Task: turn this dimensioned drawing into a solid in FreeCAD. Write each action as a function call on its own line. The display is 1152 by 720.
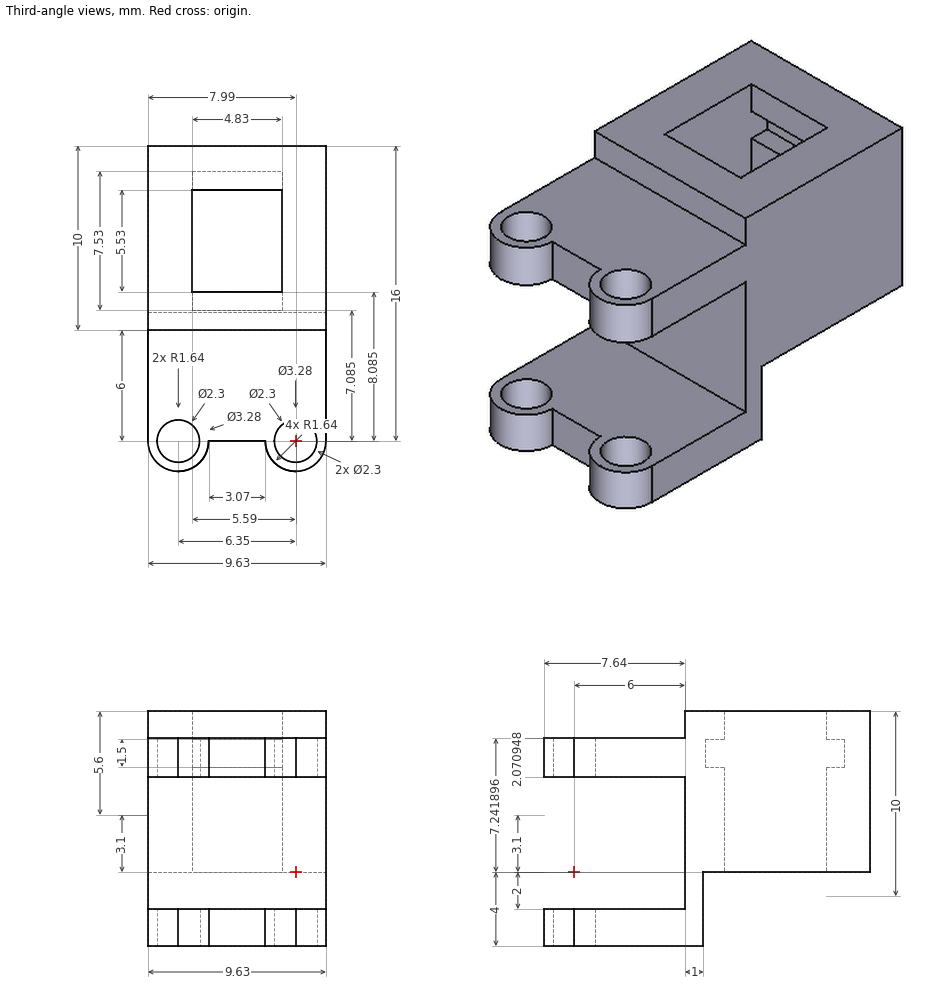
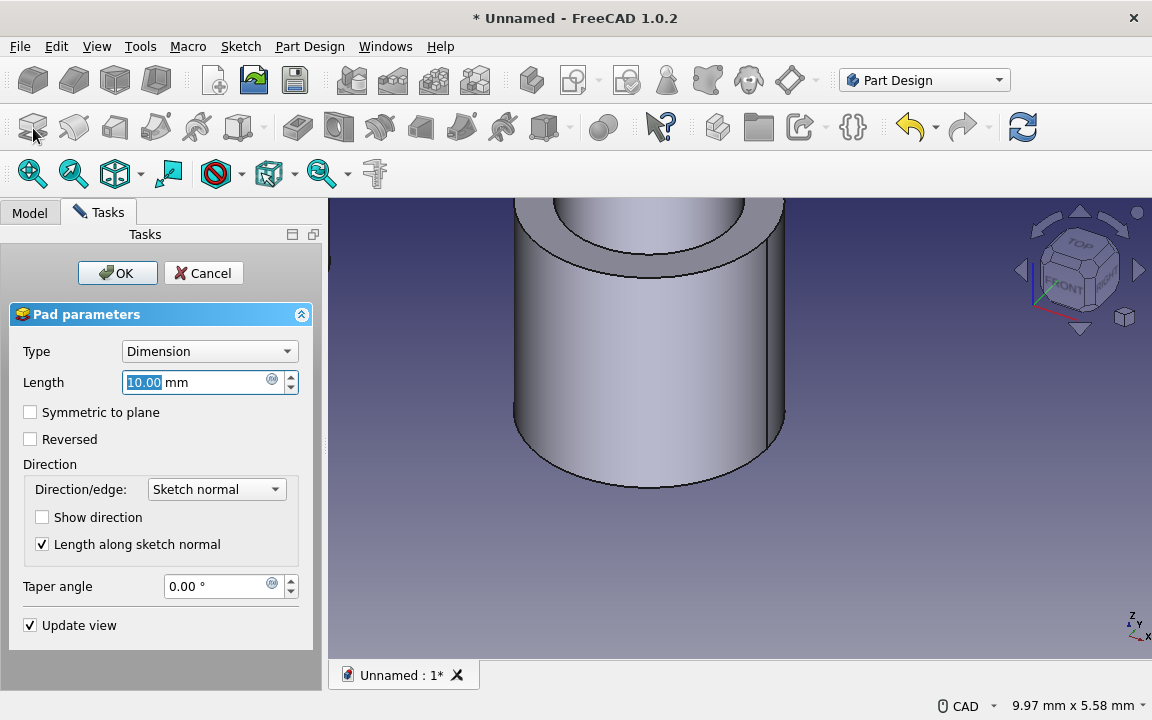
text(3.1)
key(Tab)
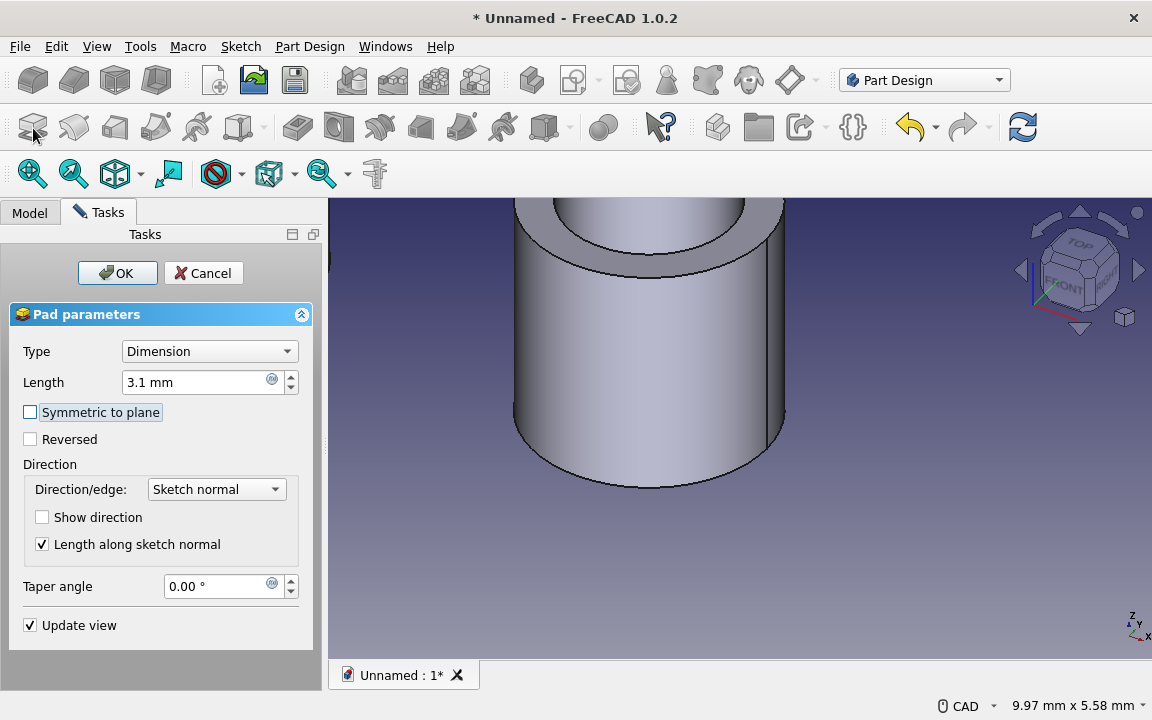
click(118, 273)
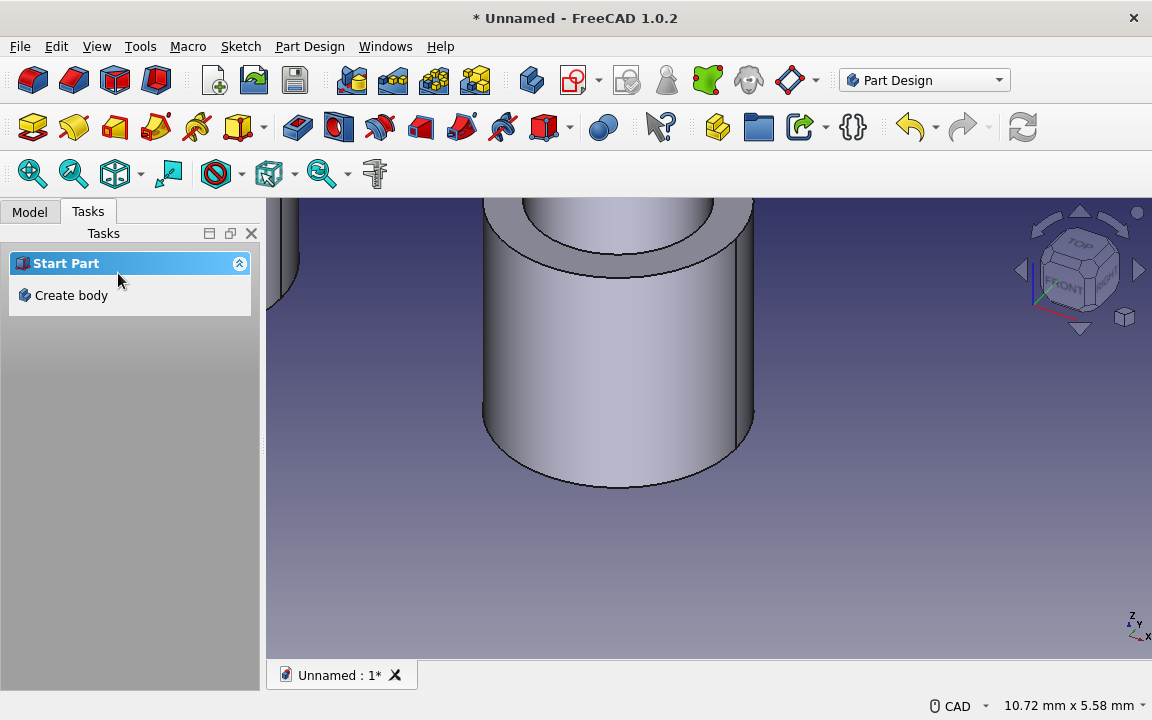
click(33, 174)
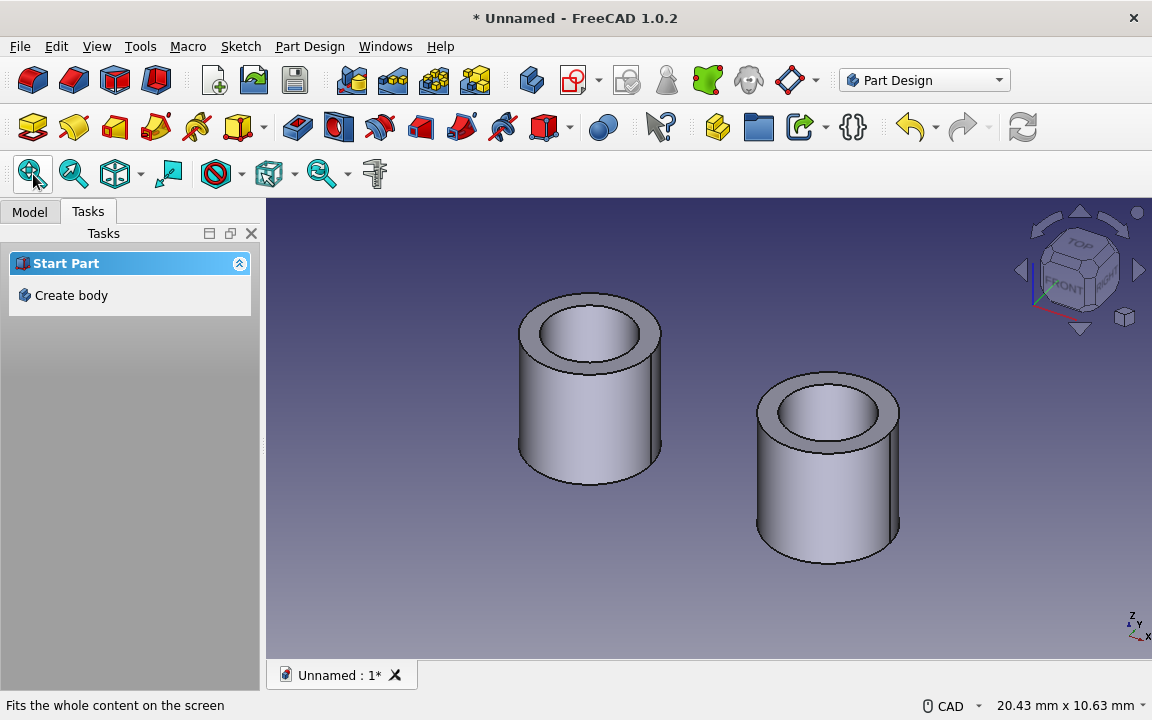
click(30, 212)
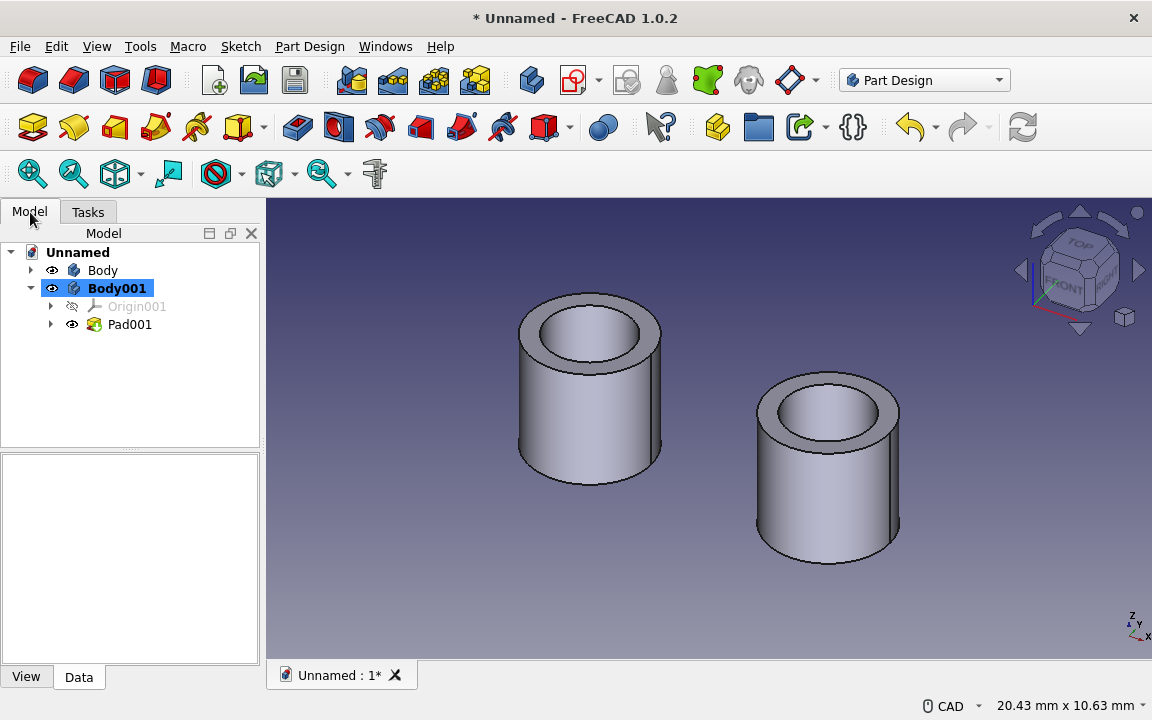
double_click(97, 270)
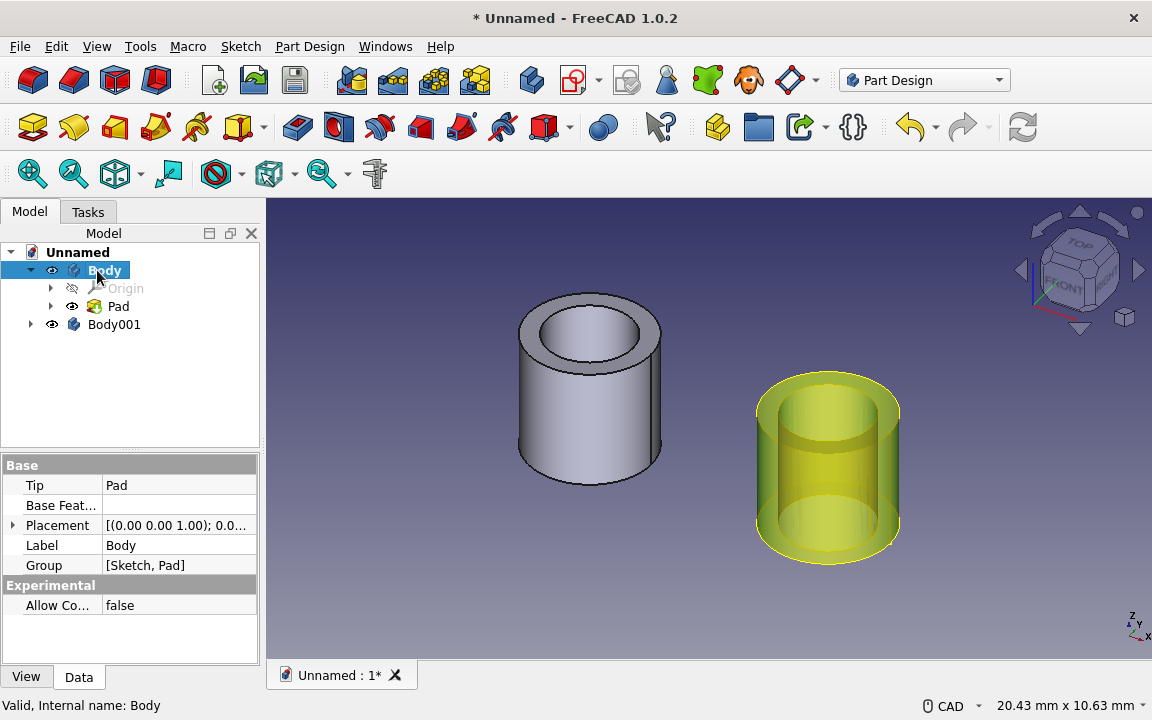
click(97, 270)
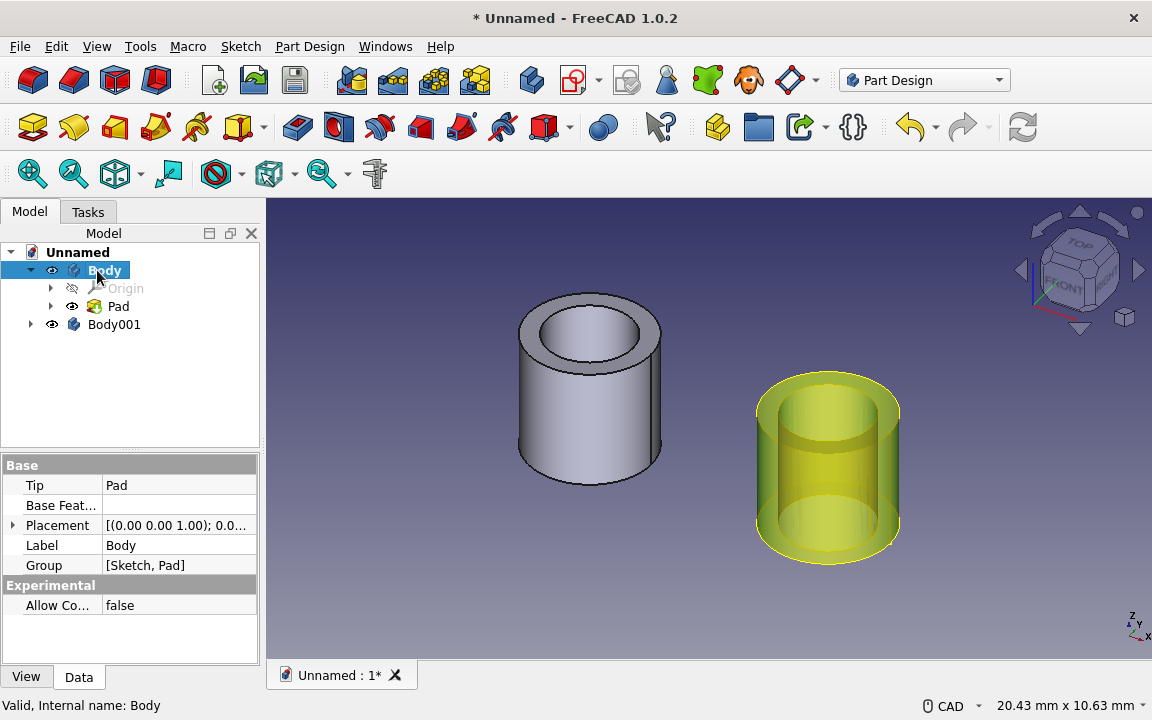
click(148, 605)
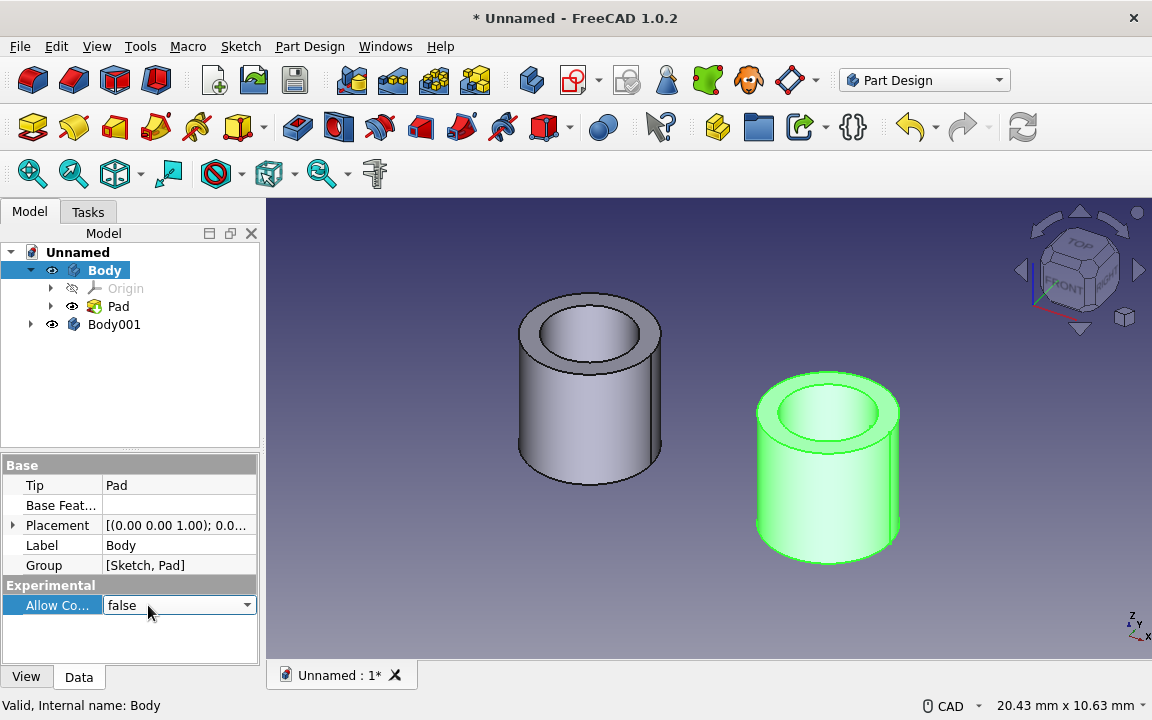
click(148, 605)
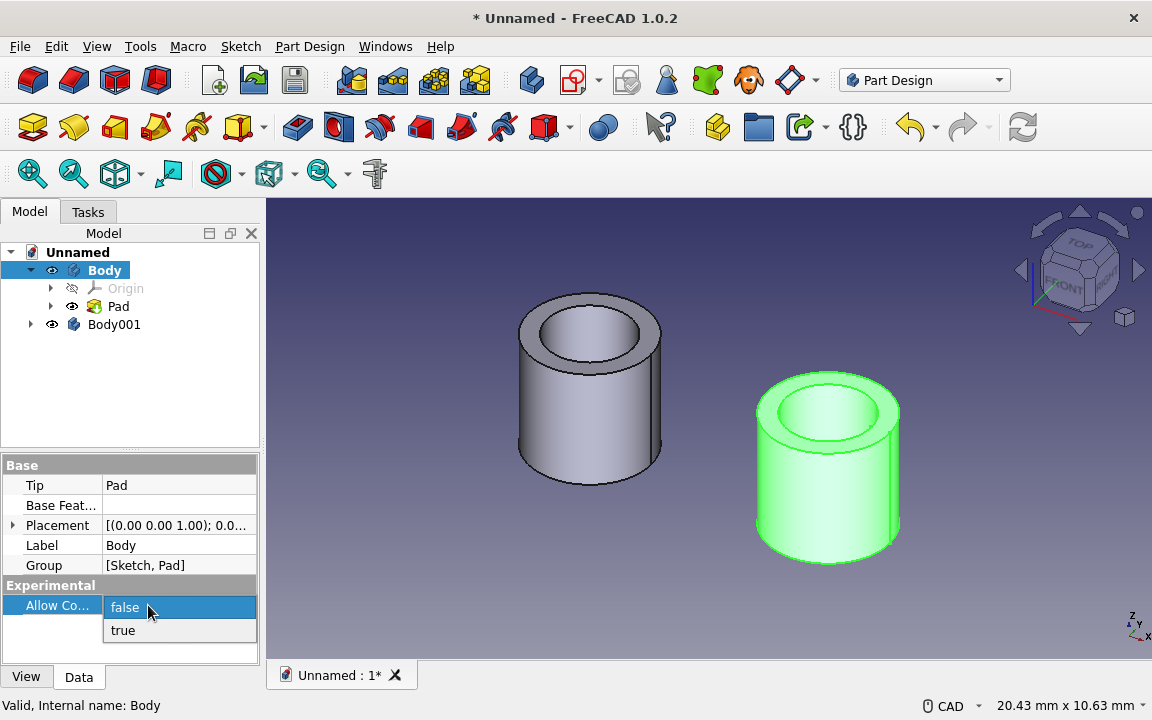
click(178, 630)
key(Return)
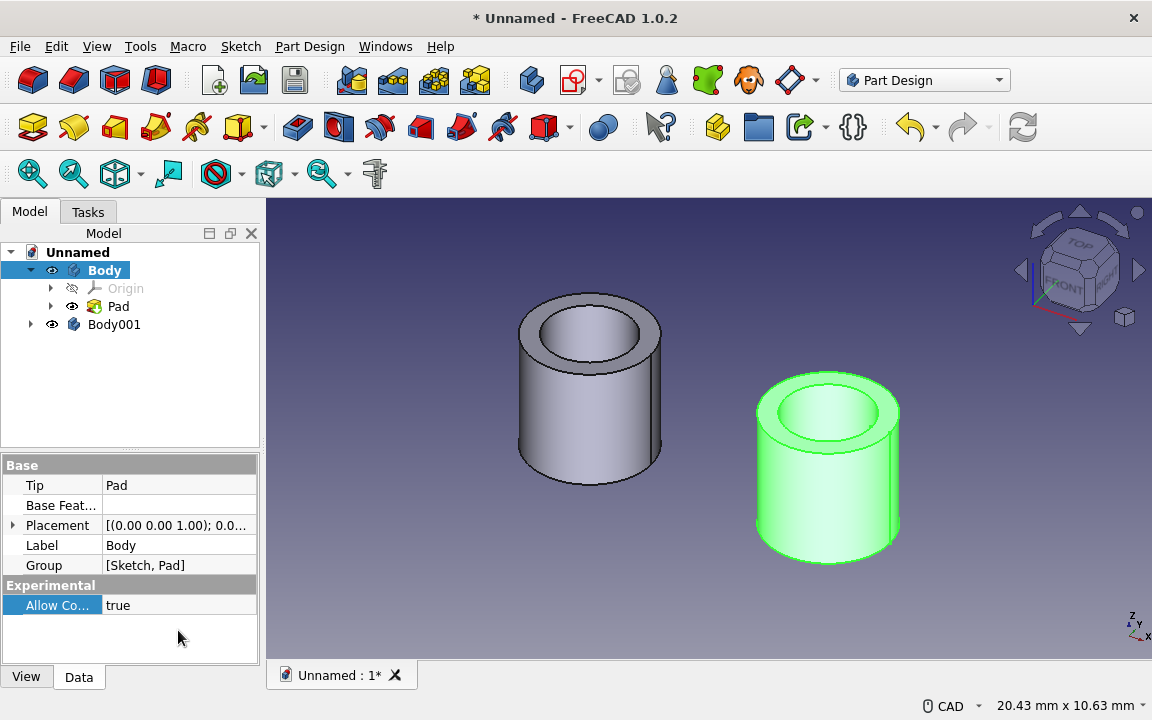
click(97, 324)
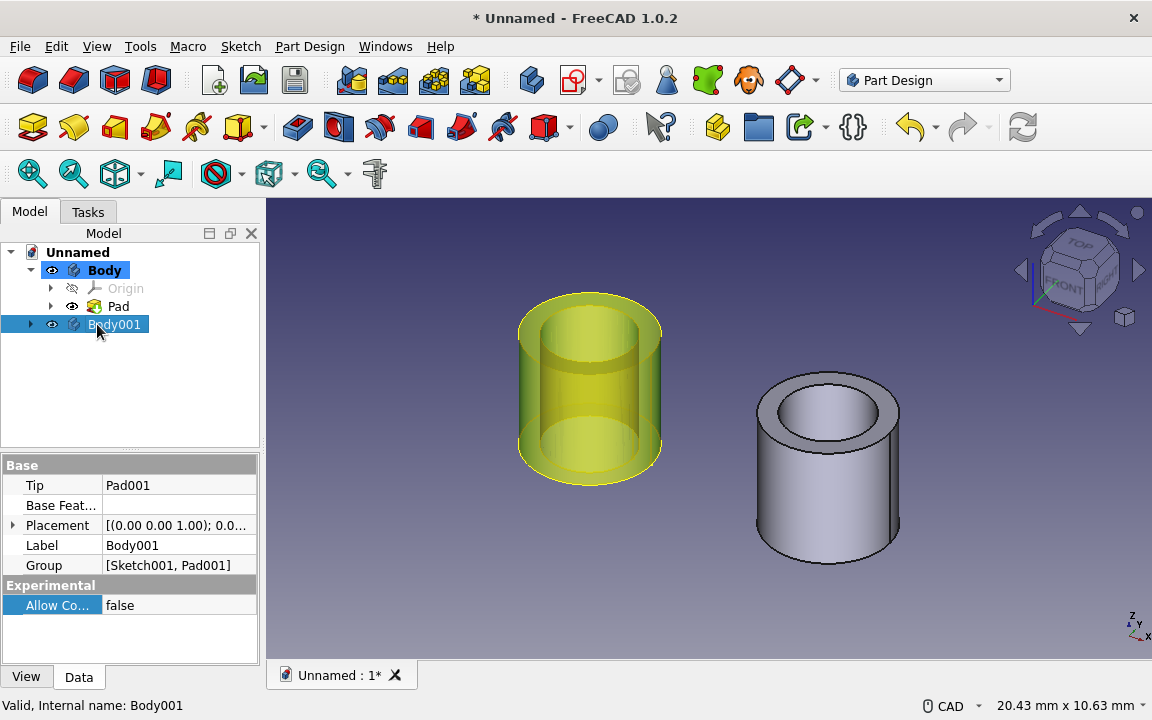
click(604, 128)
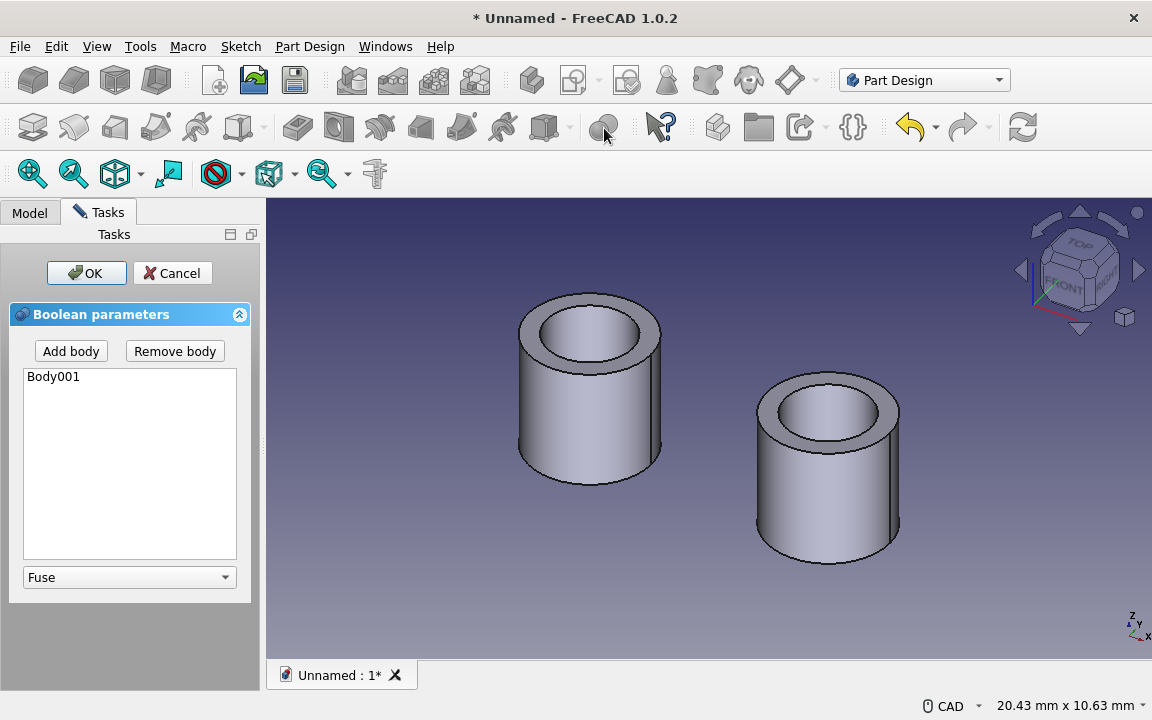
click(87, 273)